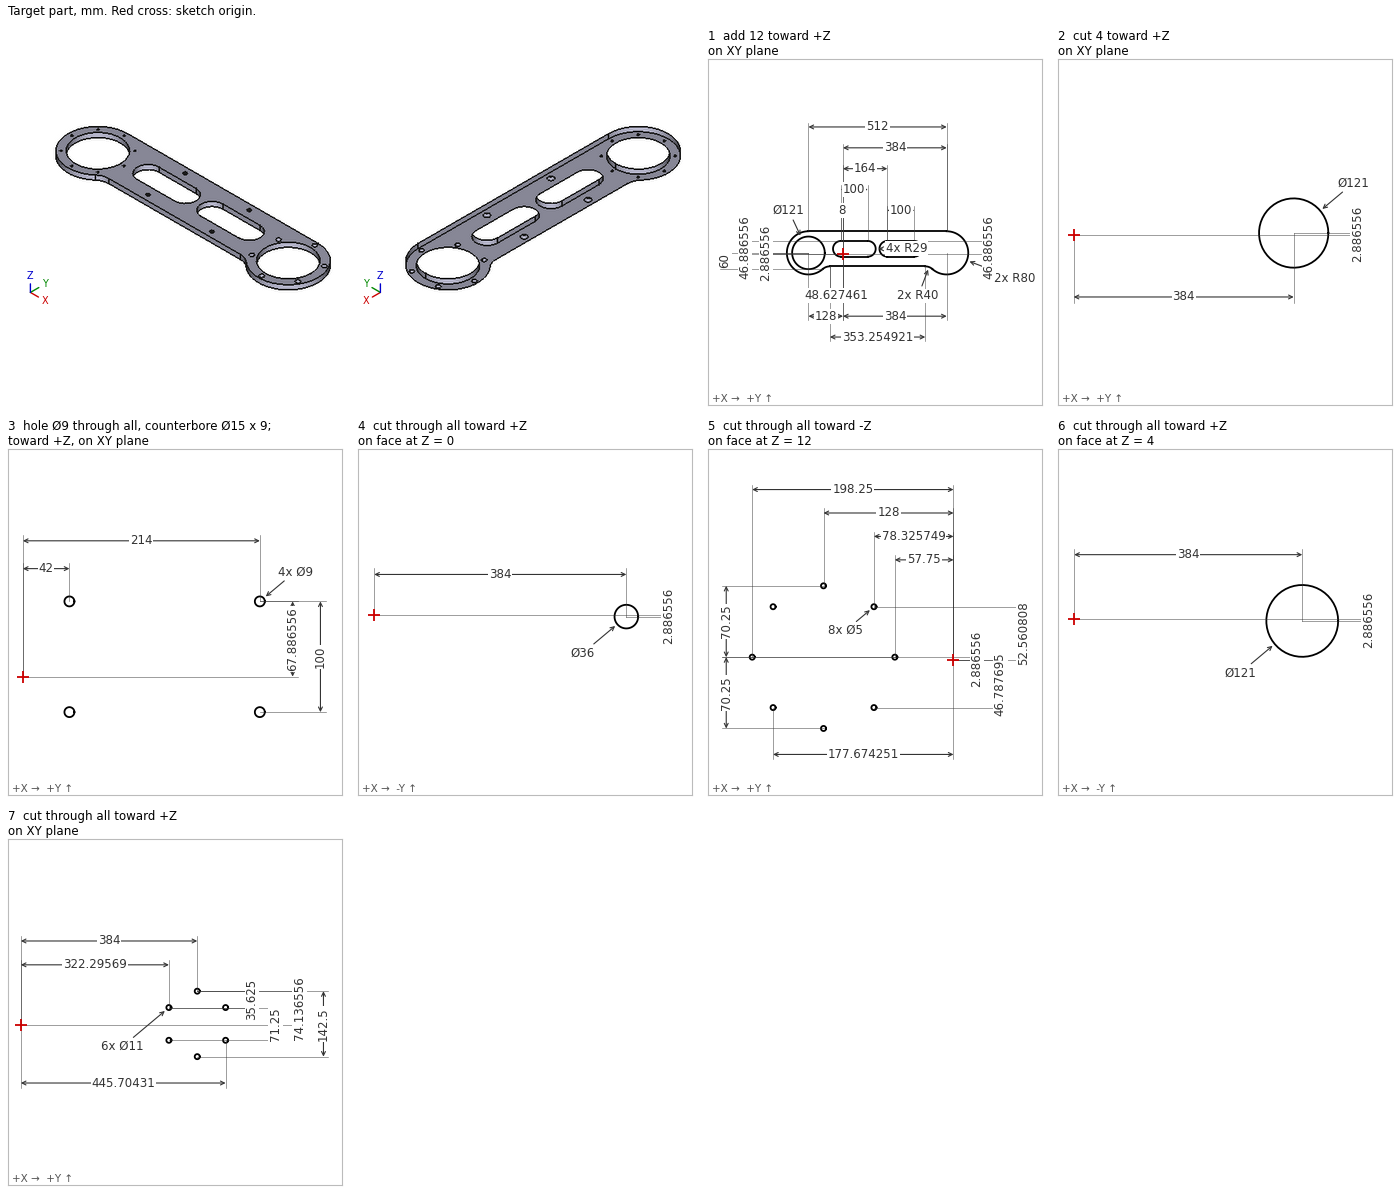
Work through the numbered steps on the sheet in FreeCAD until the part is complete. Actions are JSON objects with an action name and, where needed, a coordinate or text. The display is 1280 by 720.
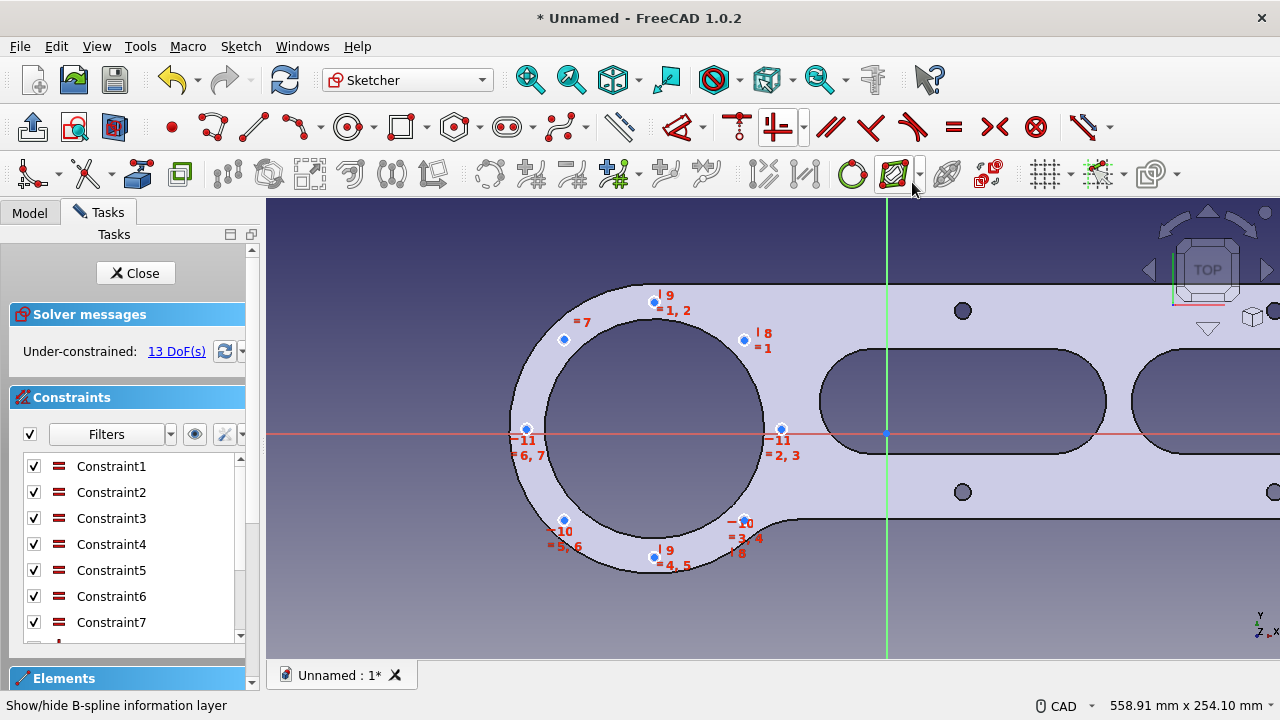
{"action": "left_click", "coordinate": [564, 520]}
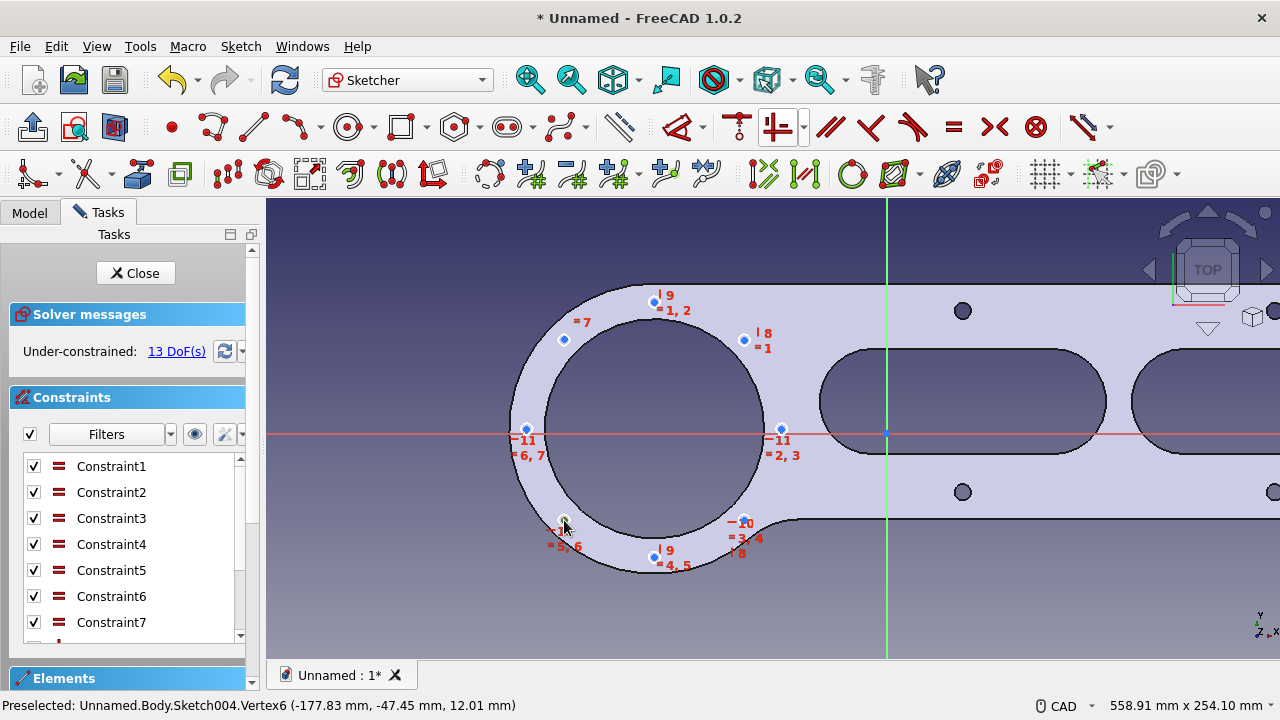
{"action": "left_click", "coordinate": [564, 340]}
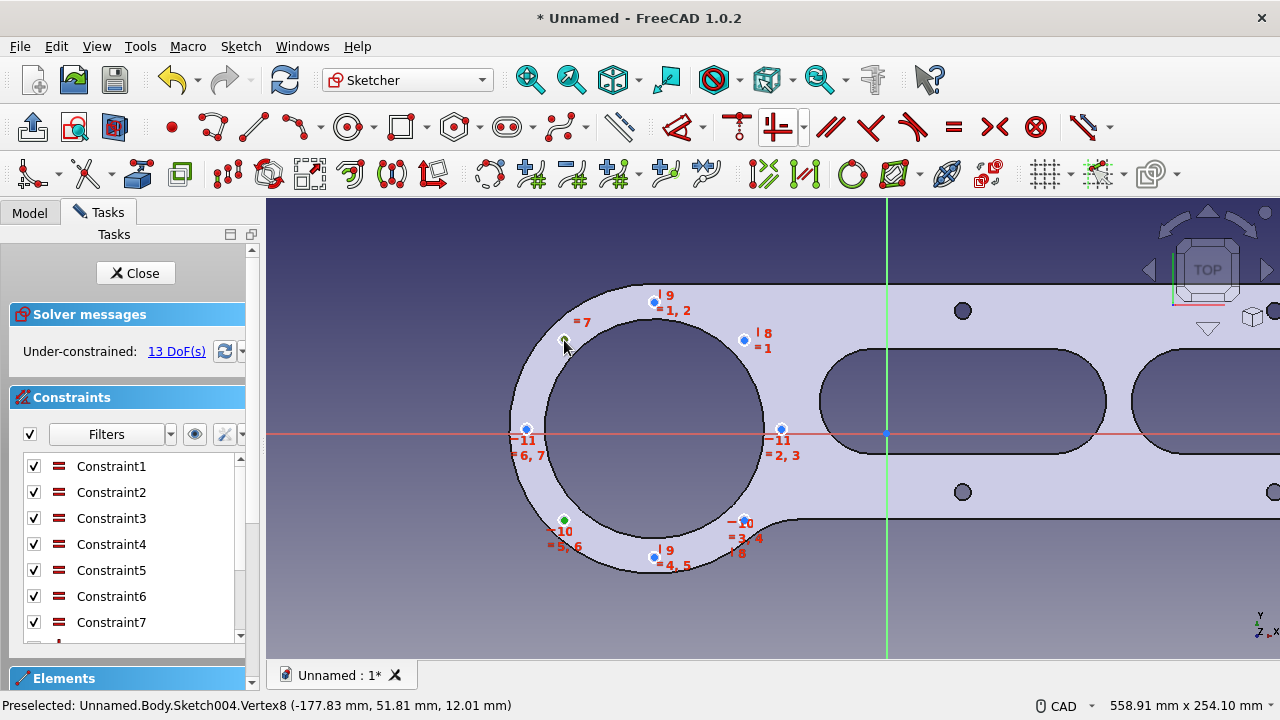
{"action": "left_click", "coordinate": [804, 128]}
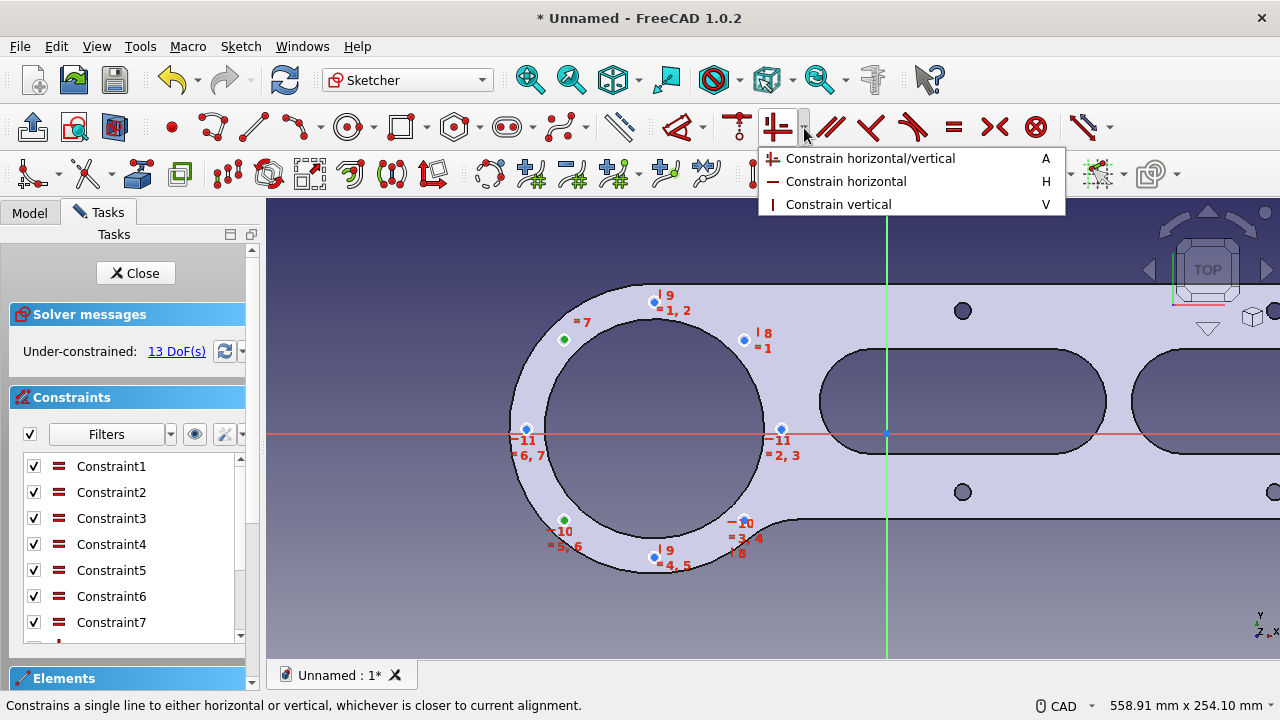
{"action": "left_click", "coordinate": [912, 204]}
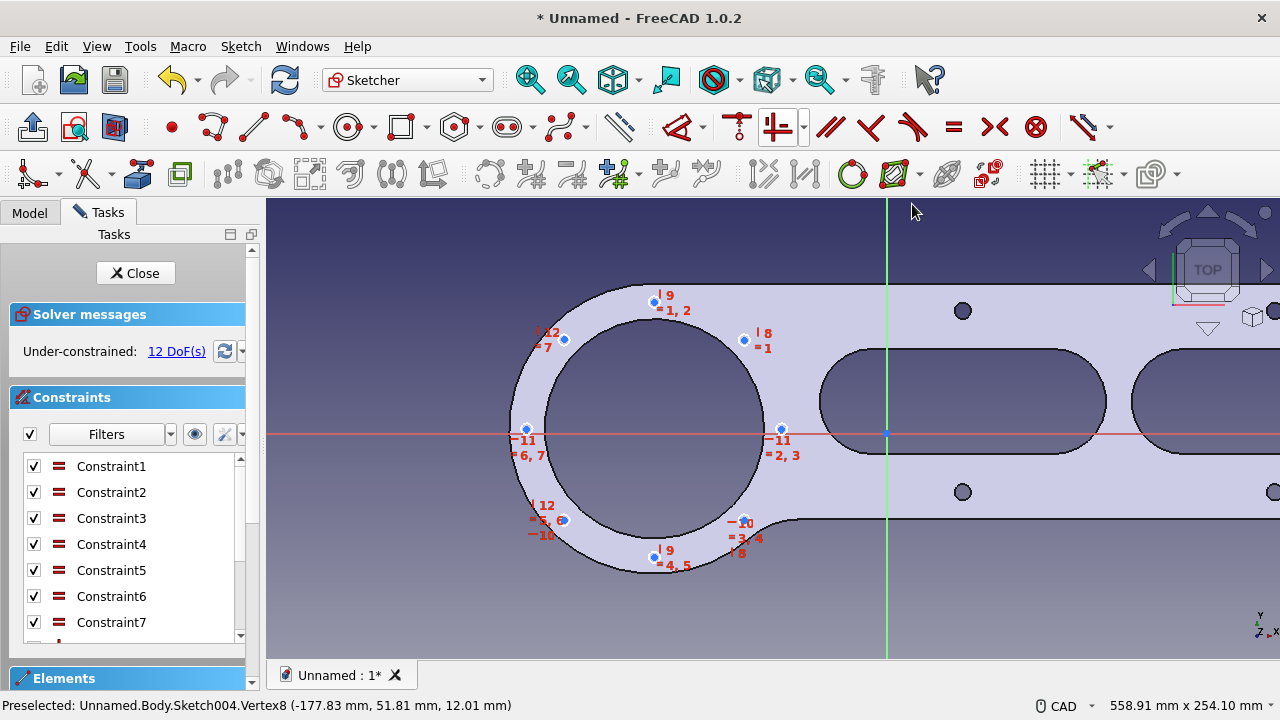
{"action": "left_click", "coordinate": [744, 340]}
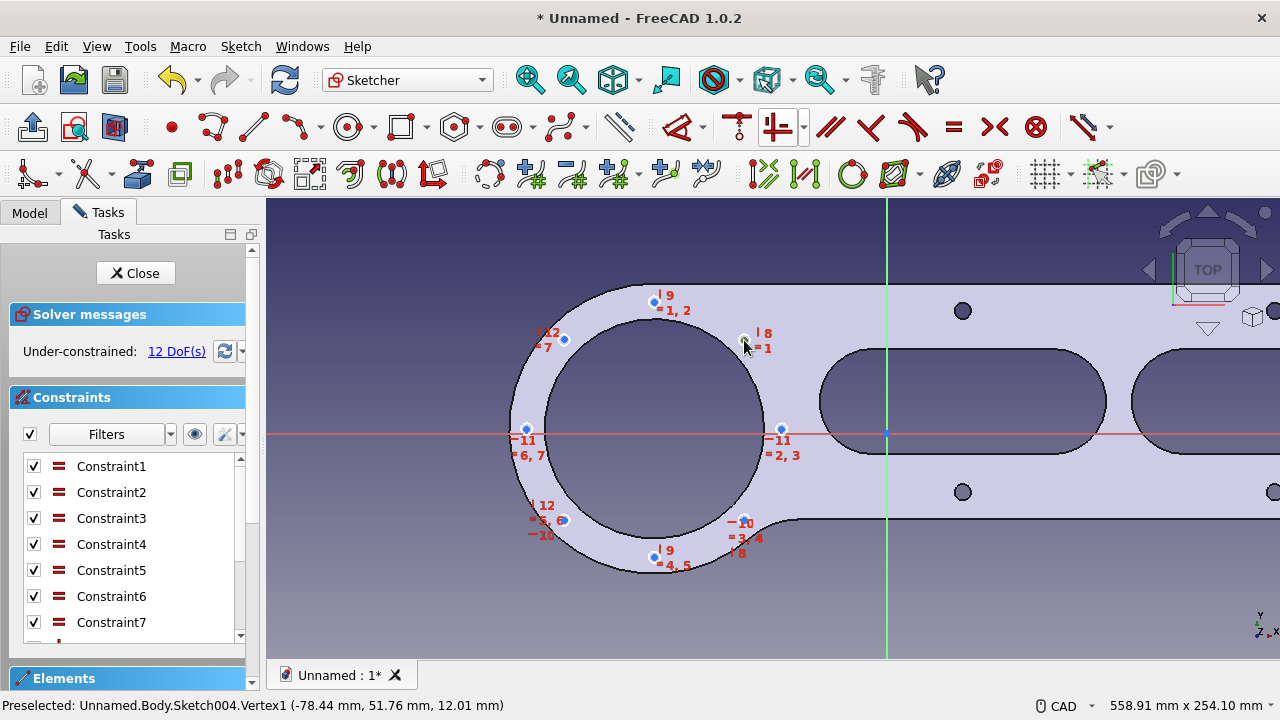
{"action": "left_click", "coordinate": [564, 340]}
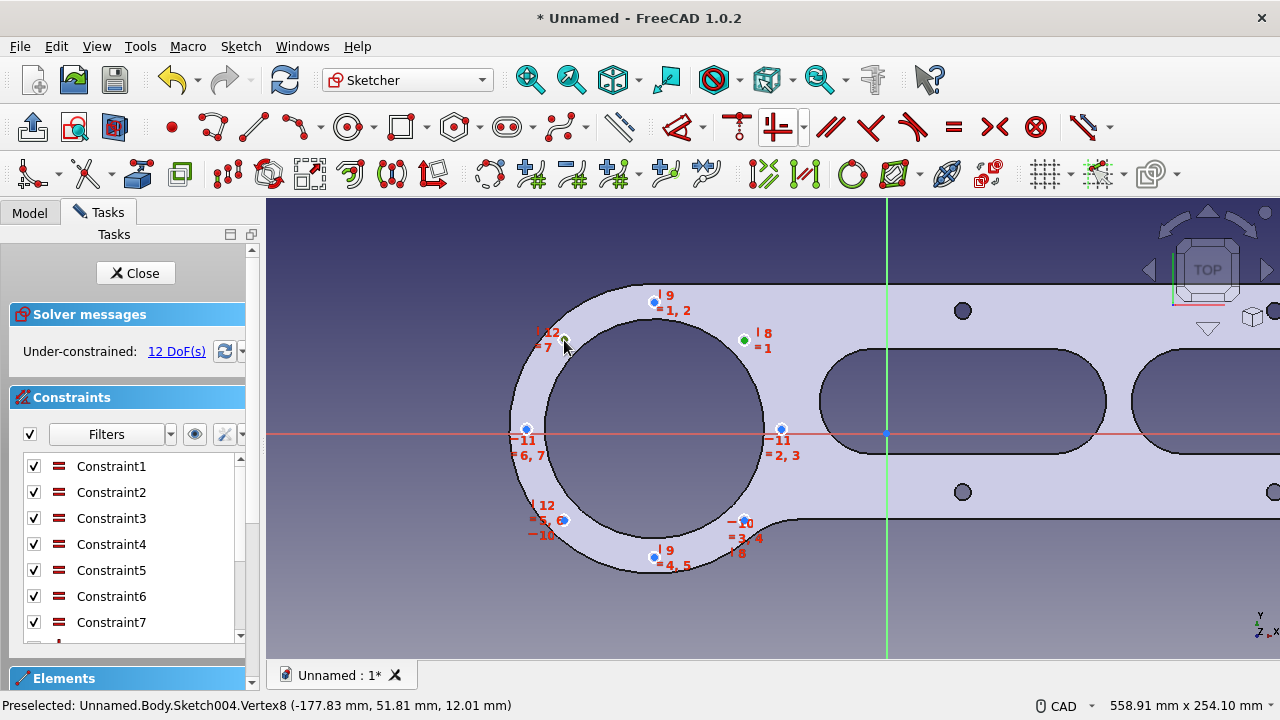
{"action": "left_click", "coordinate": [804, 128]}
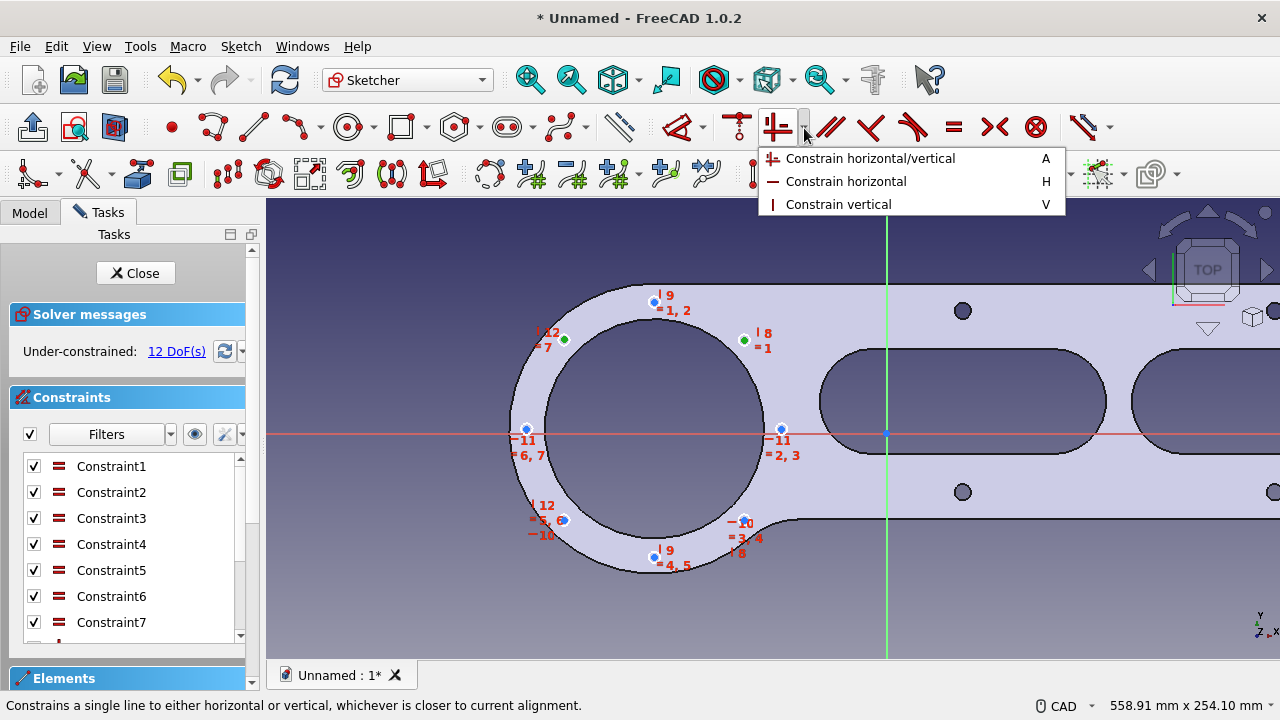
{"action": "left_click", "coordinate": [912, 182]}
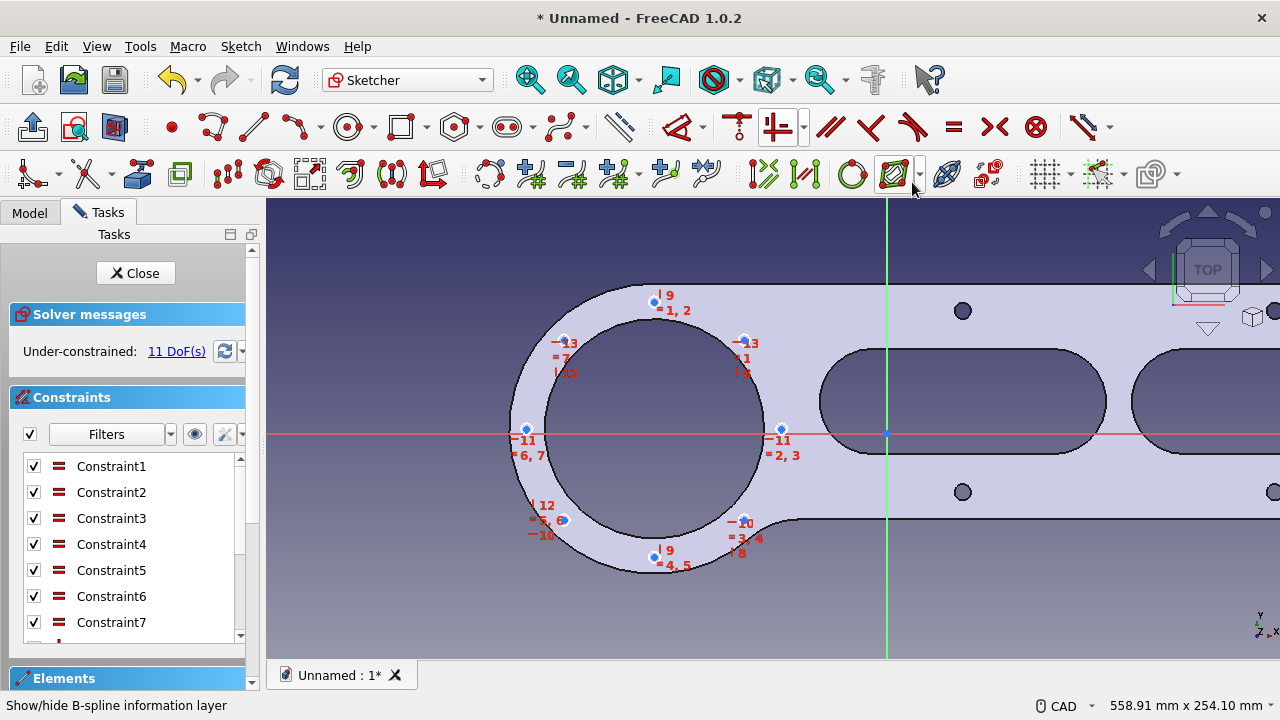
{"action": "left_click", "coordinate": [676, 128]}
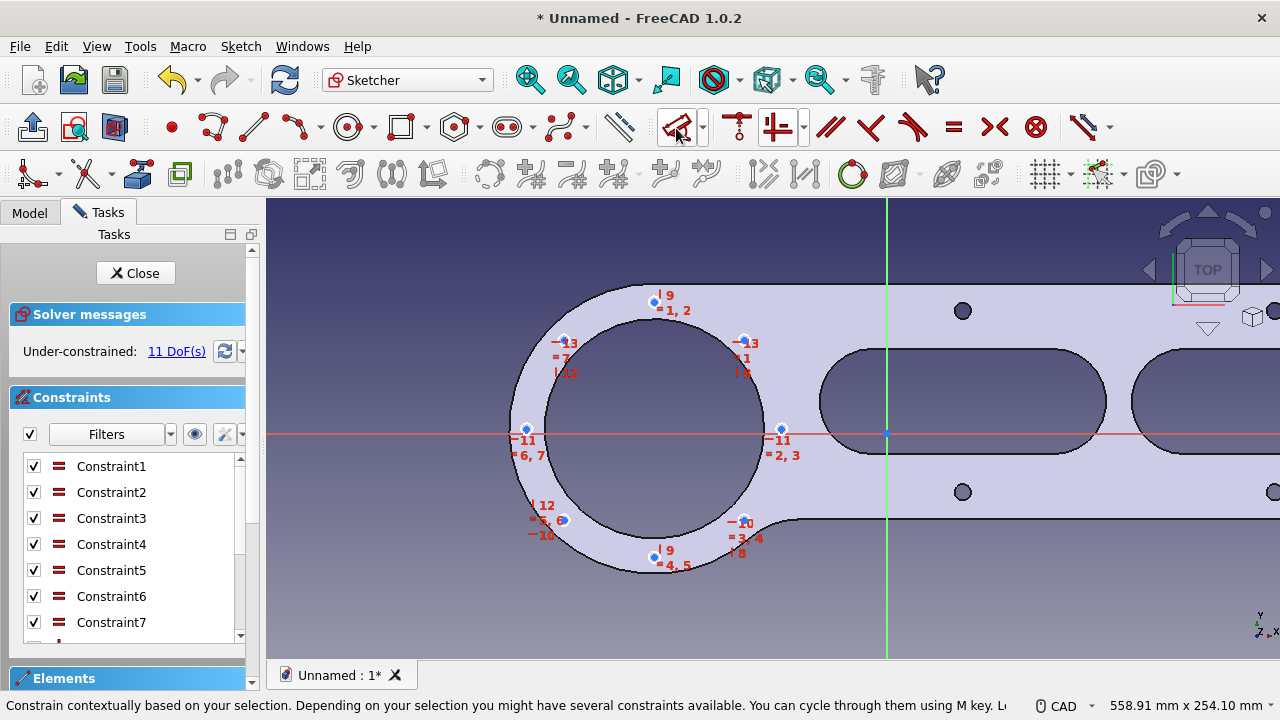
{"action": "scroll", "coordinate": [739, 340], "scroll_direction": "up", "scroll_amount": 8}